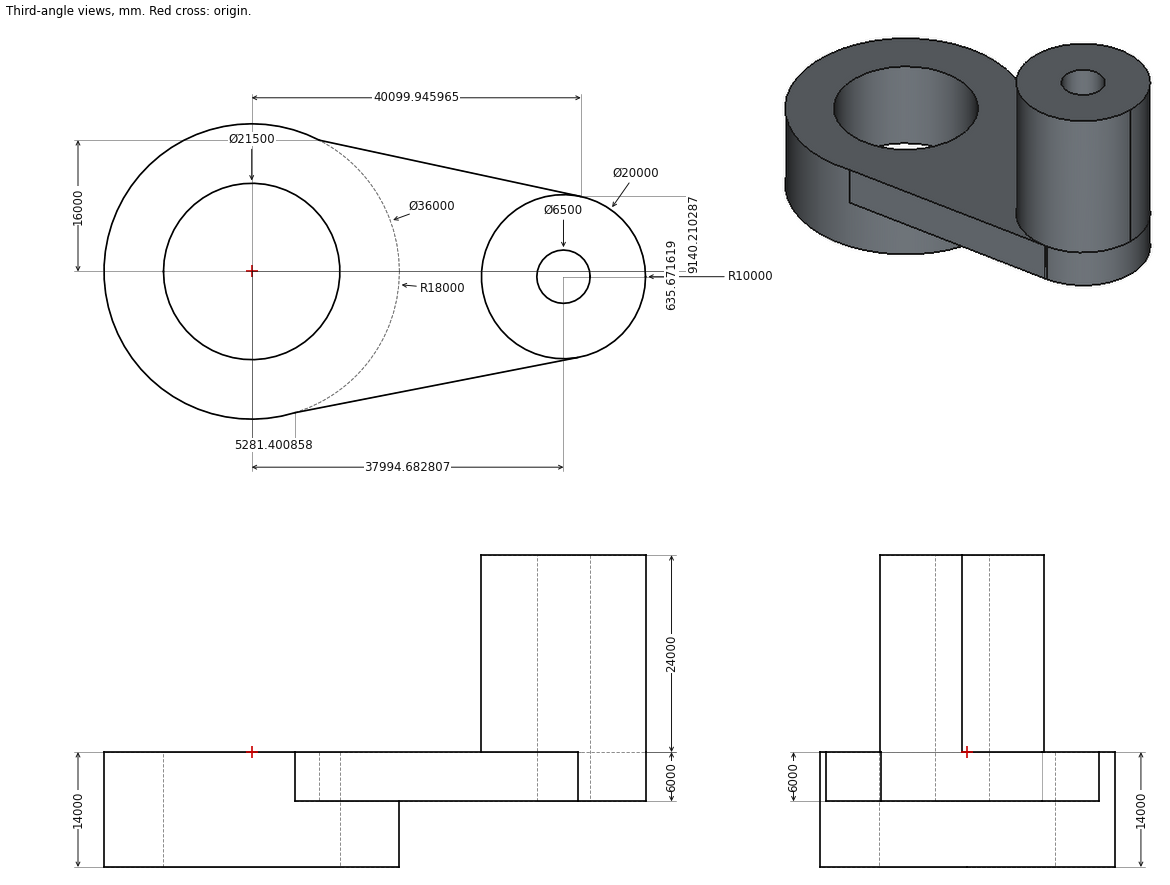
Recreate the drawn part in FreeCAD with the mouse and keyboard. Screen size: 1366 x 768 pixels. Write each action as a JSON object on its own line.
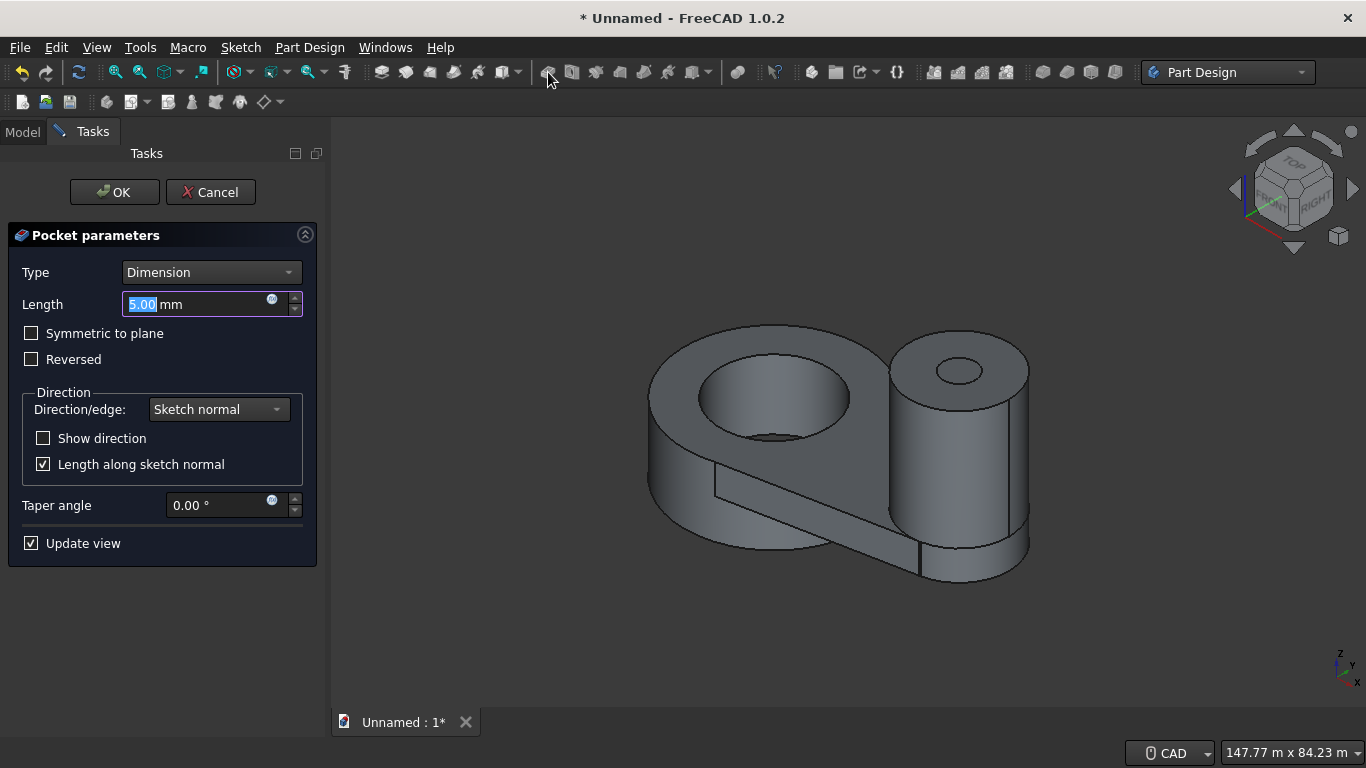
{"action": "left_click", "coordinate": [212, 272]}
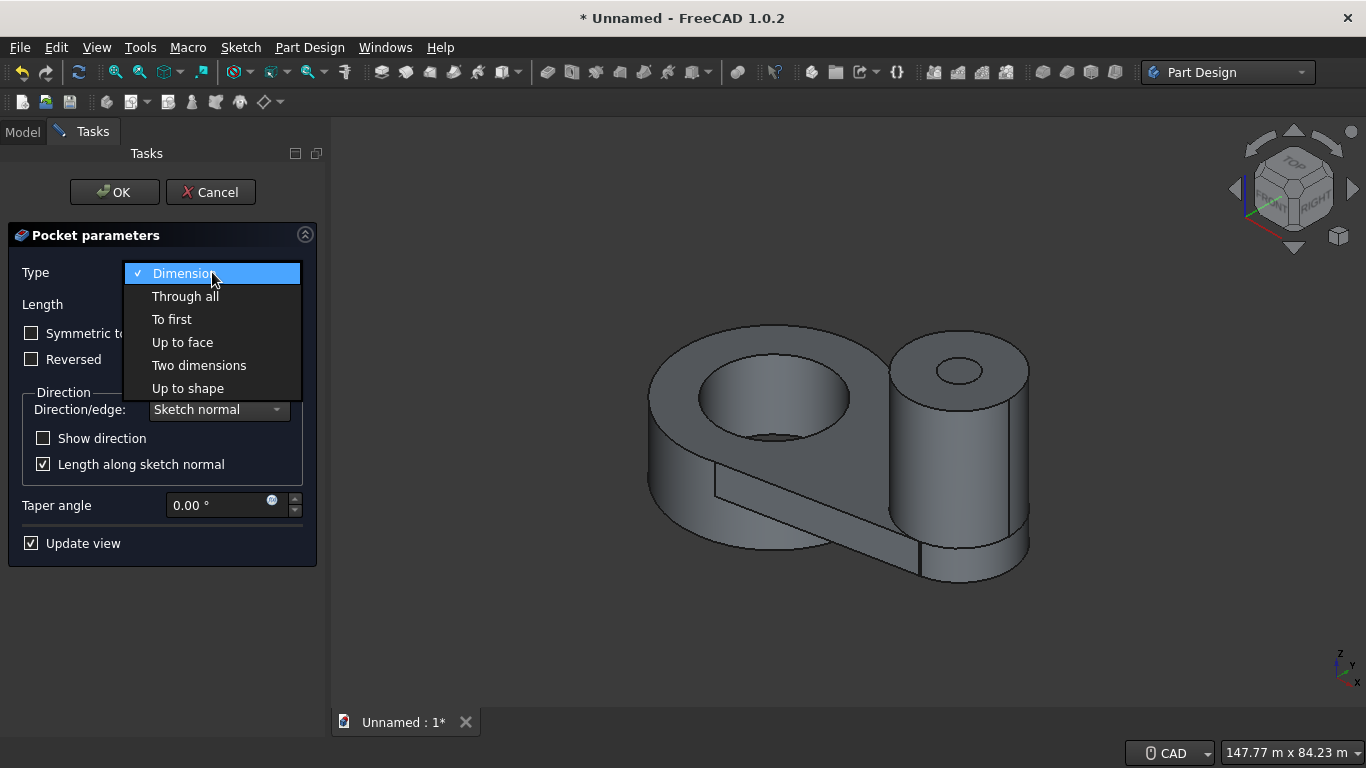
{"action": "left_click", "coordinate": [212, 296]}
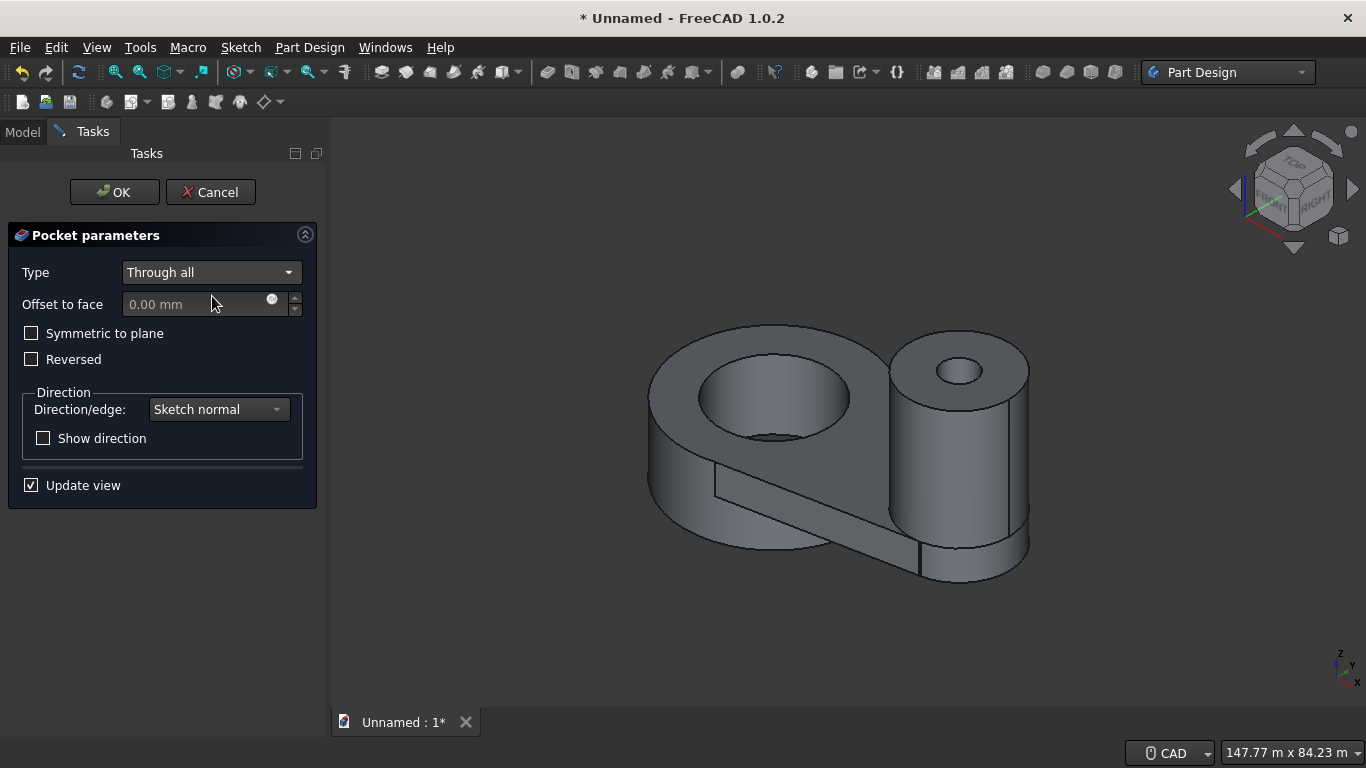
{"action": "left_click", "coordinate": [115, 192]}